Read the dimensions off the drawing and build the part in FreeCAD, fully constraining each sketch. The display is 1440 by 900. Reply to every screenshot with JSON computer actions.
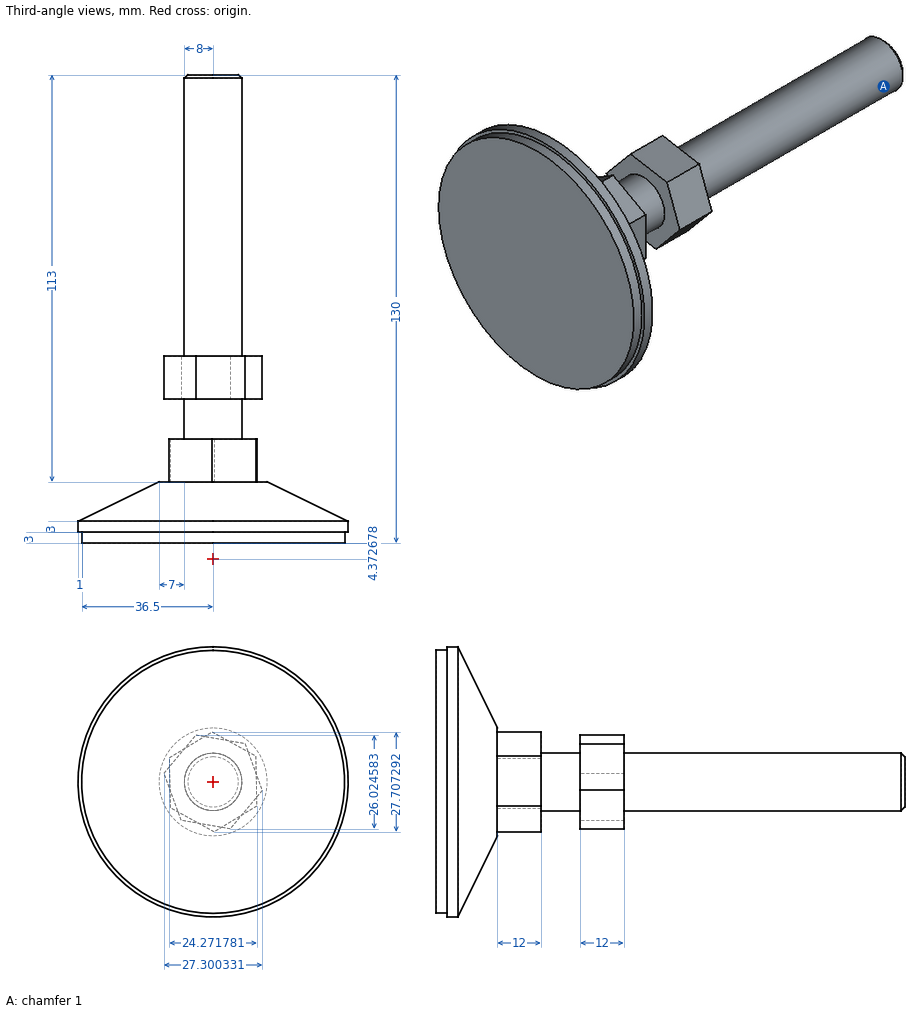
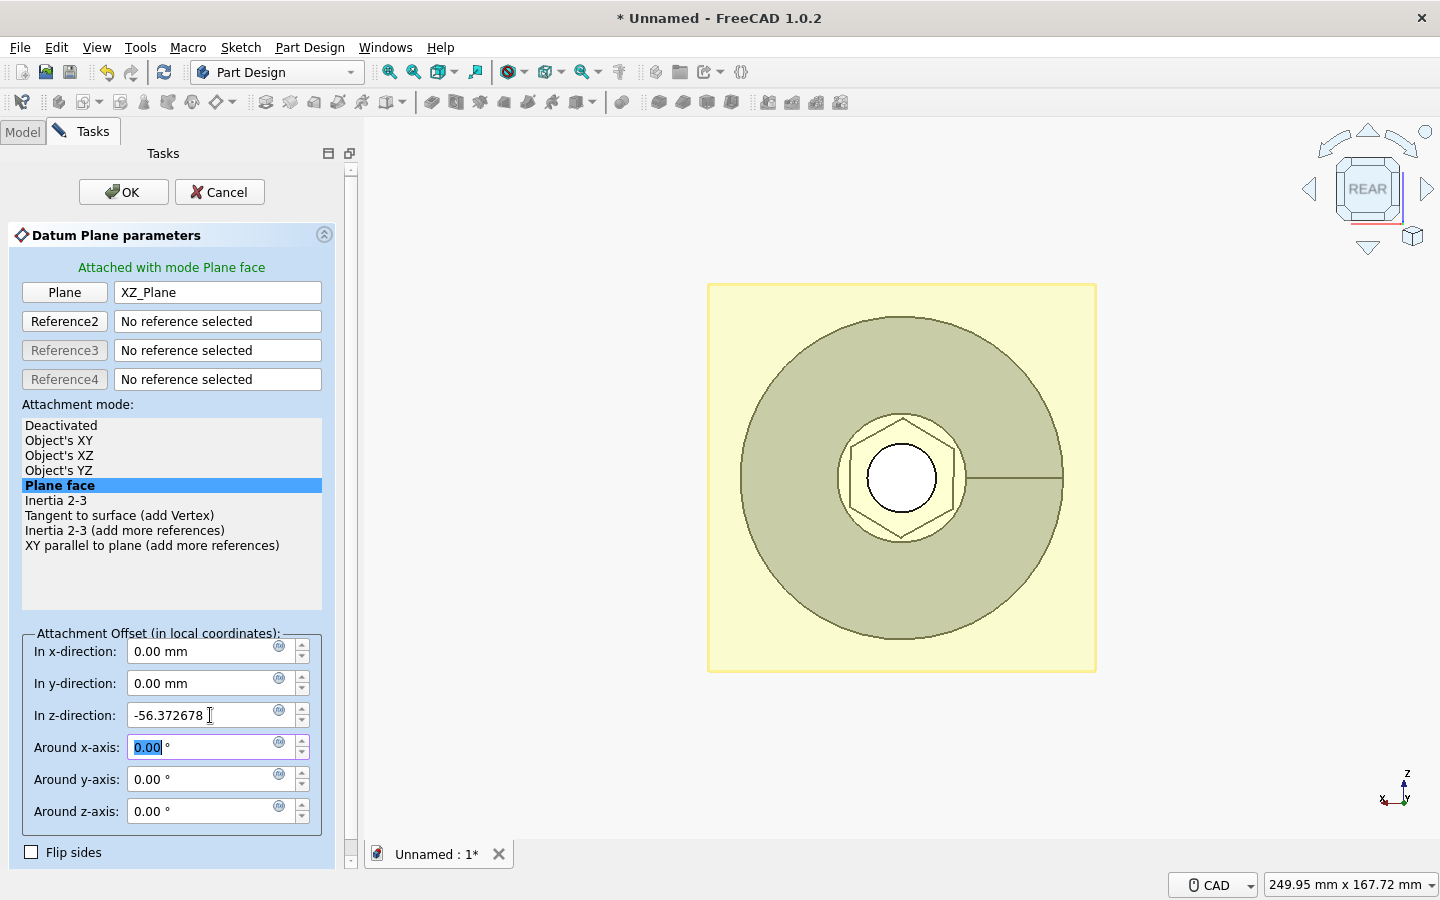
{"action": "left_click", "coordinate": [124, 192]}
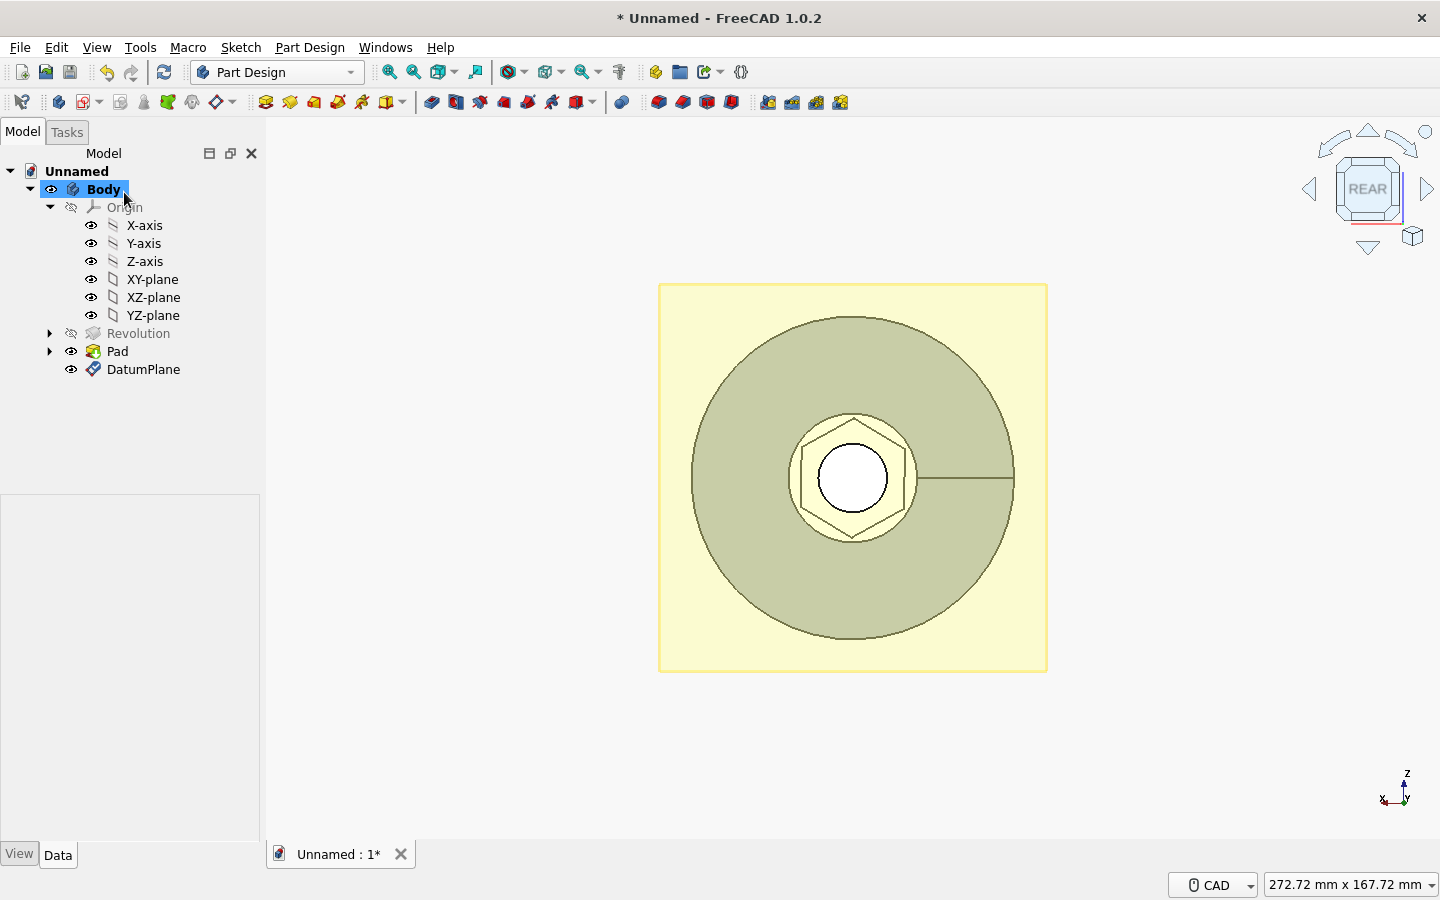
{"action": "left_click", "coordinate": [116, 369]}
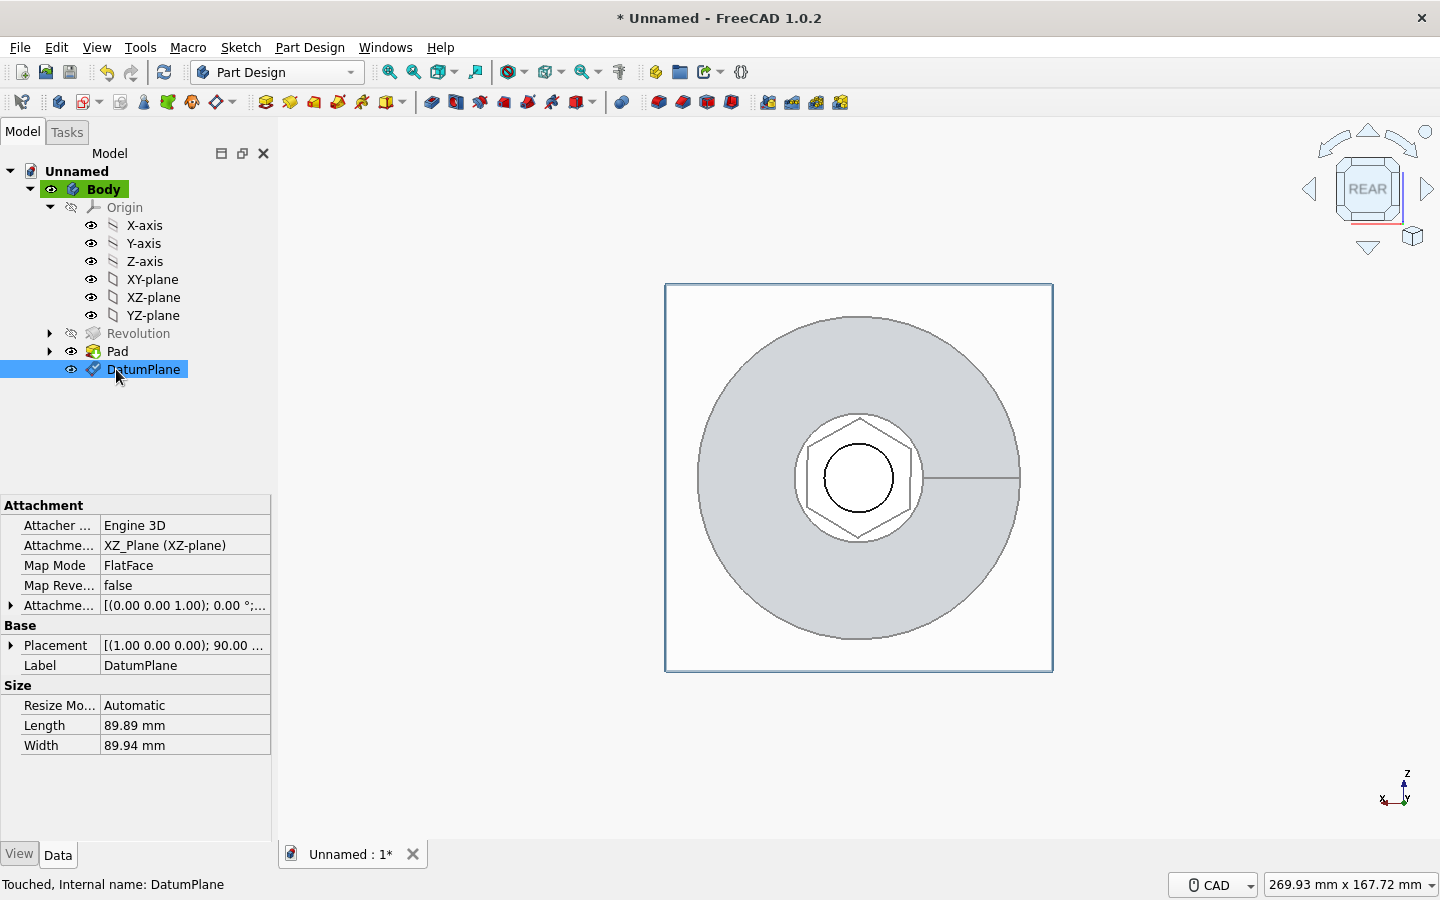
{"action": "left_click", "coordinate": [84, 102]}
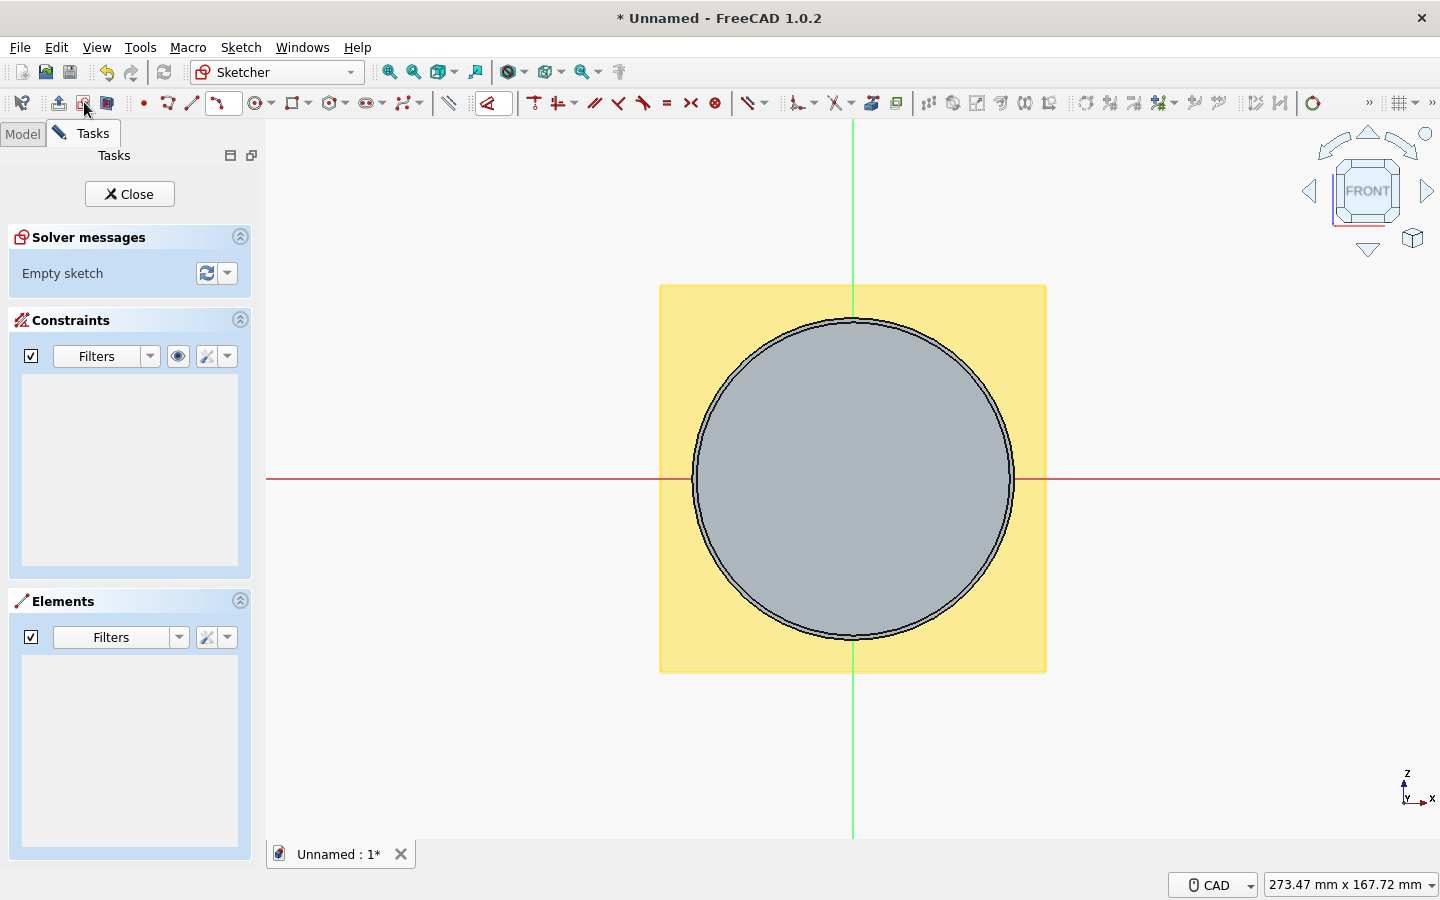
{"action": "left_click", "coordinate": [108, 104]}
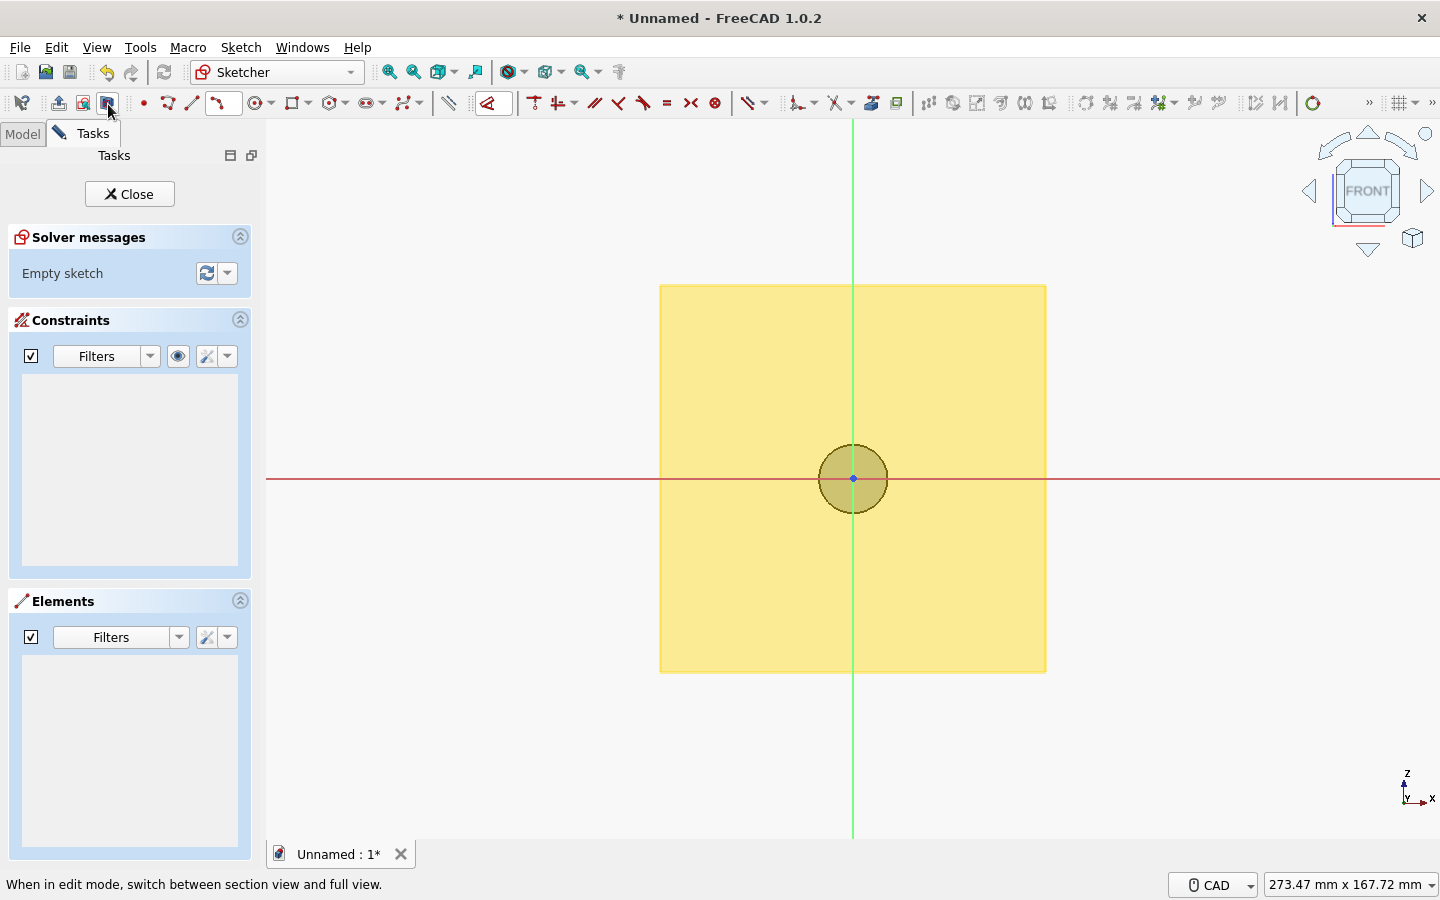
{"action": "scroll", "coordinate": [876, 479], "scroll_direction": "up", "scroll_amount": 7}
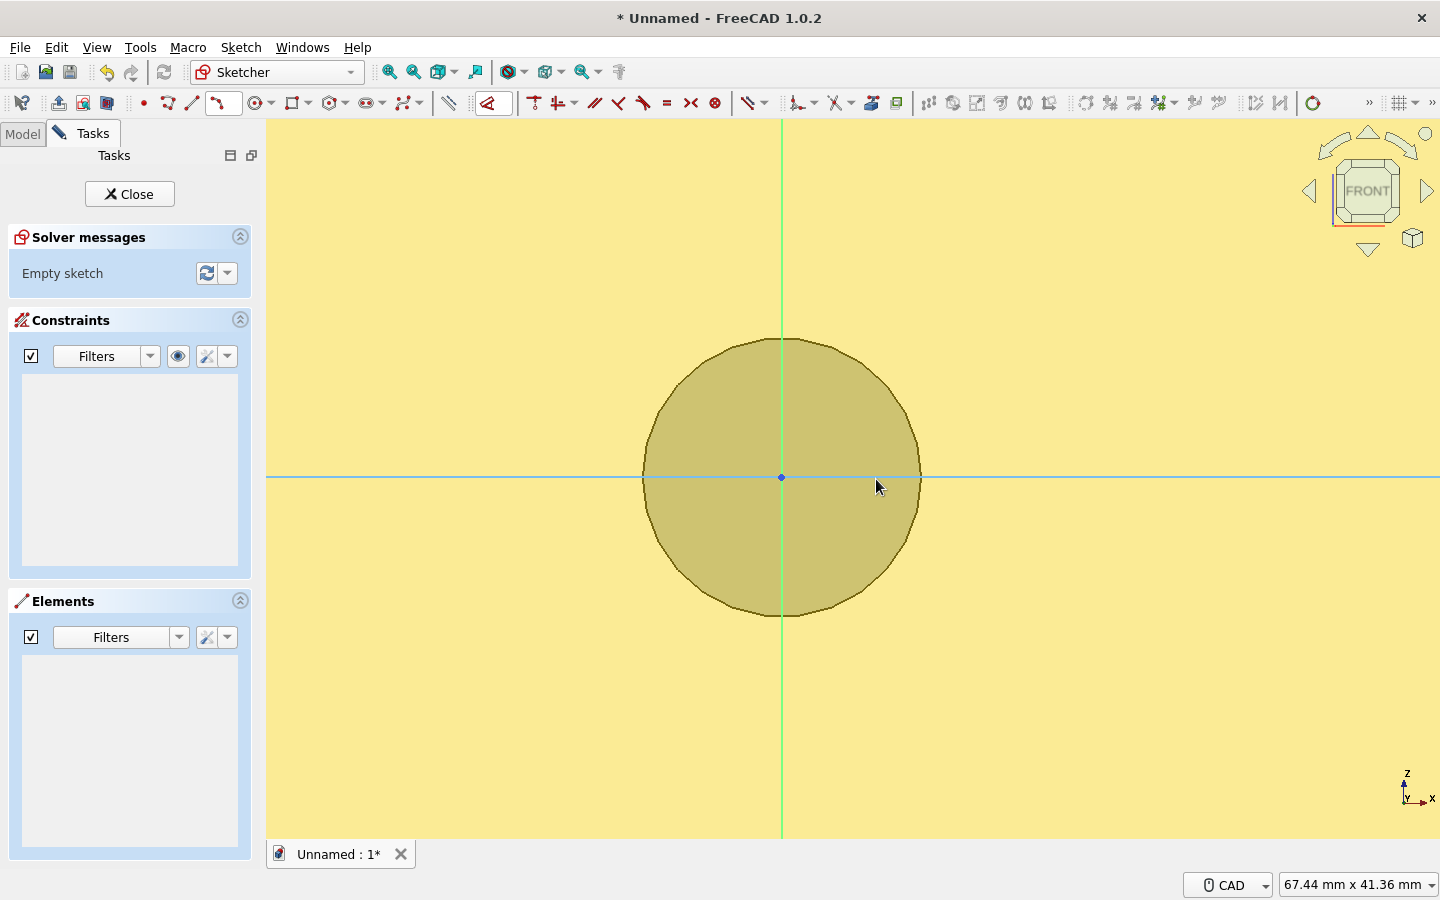
{"action": "left_click", "coordinate": [330, 104]}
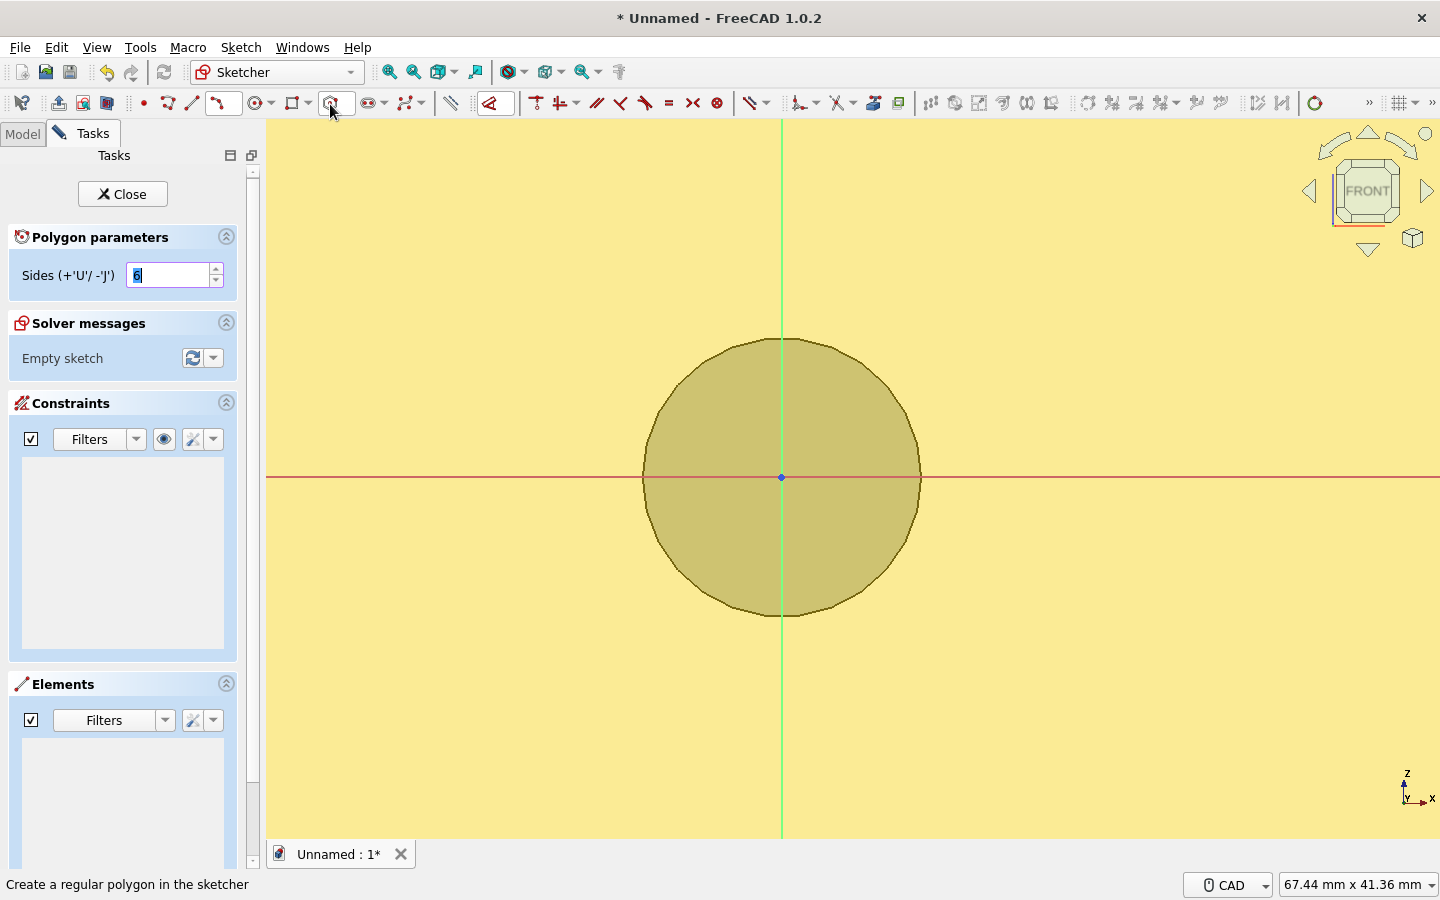
{"action": "left_click", "coordinate": [782, 477]}